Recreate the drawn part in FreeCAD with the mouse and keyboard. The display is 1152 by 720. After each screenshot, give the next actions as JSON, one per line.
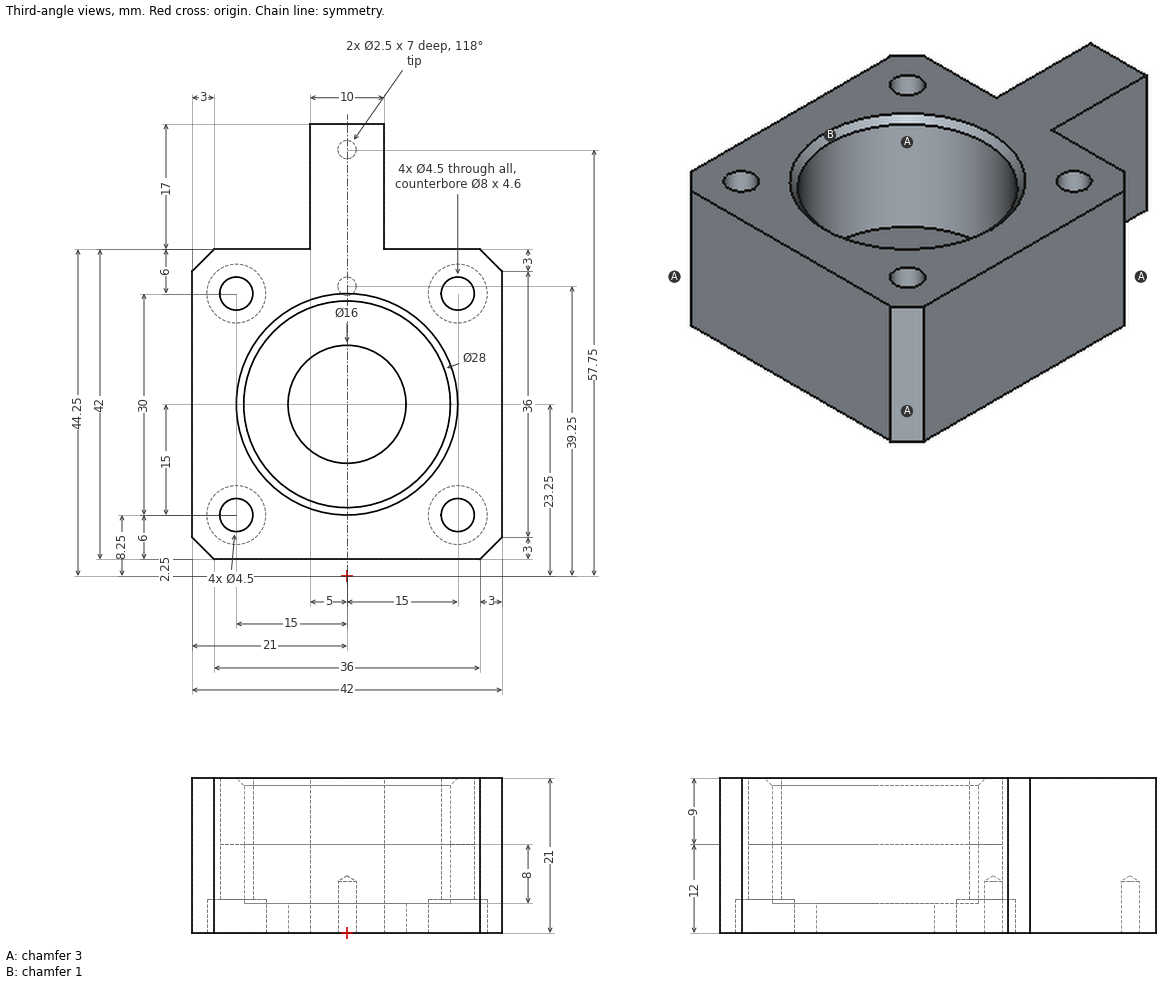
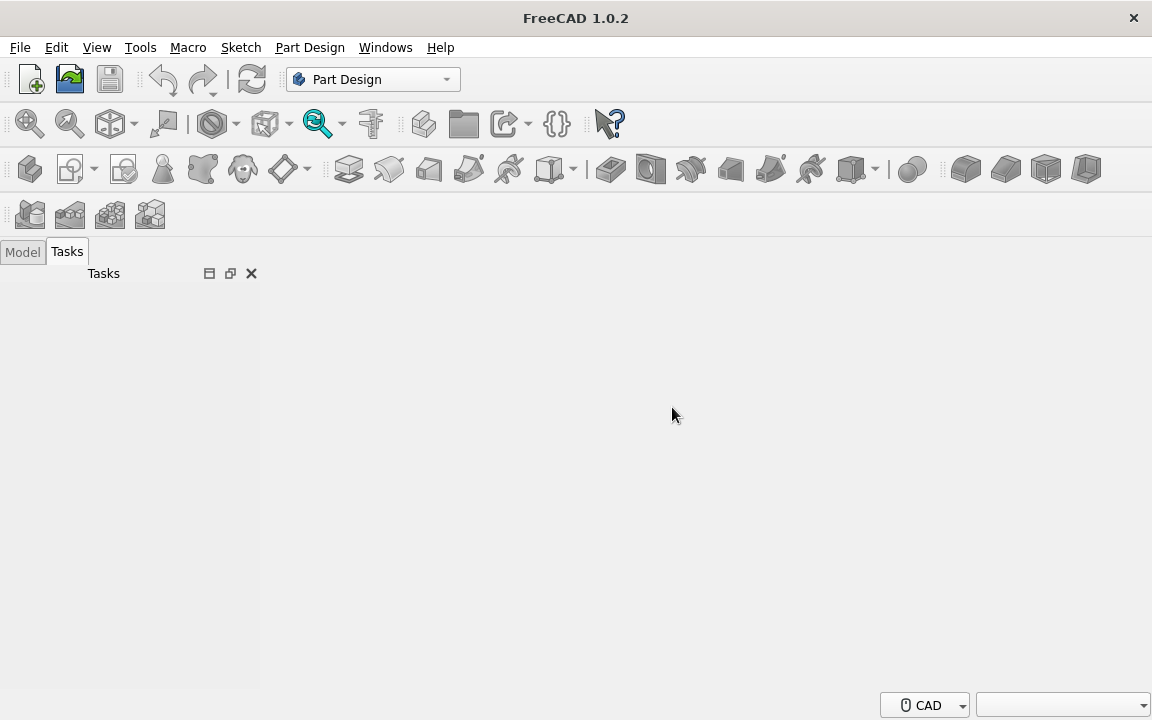
{"action": "left_click", "coordinate": [30, 80]}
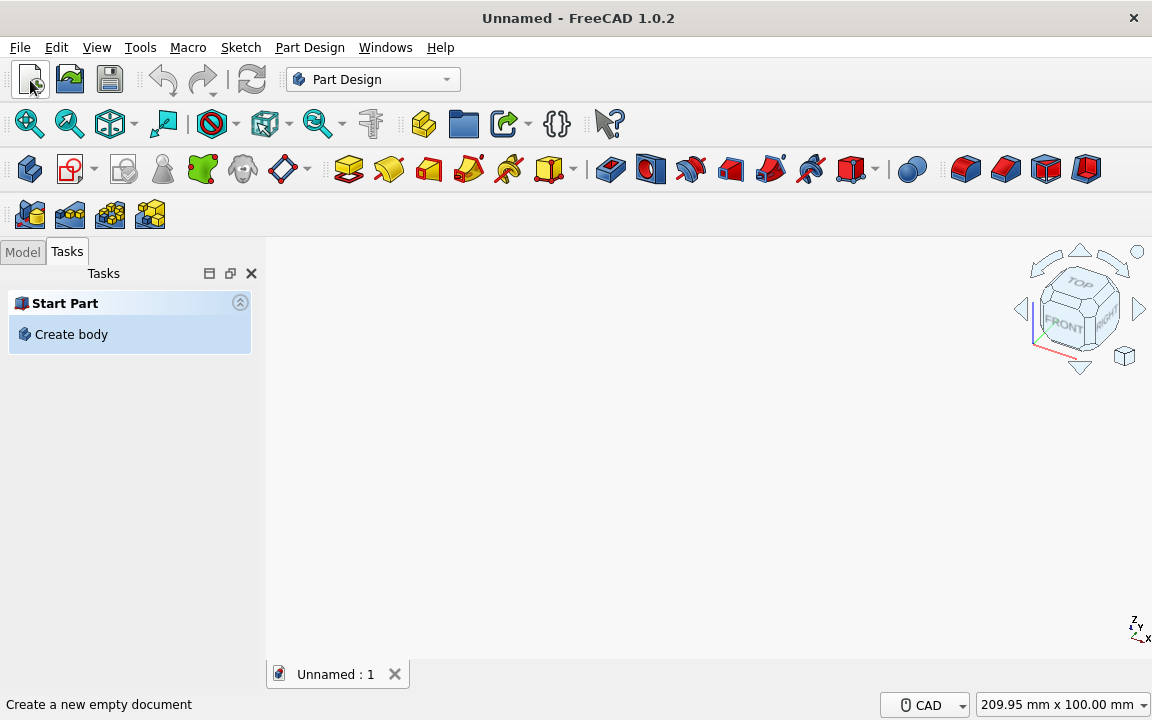
{"action": "left_click", "coordinate": [70, 170]}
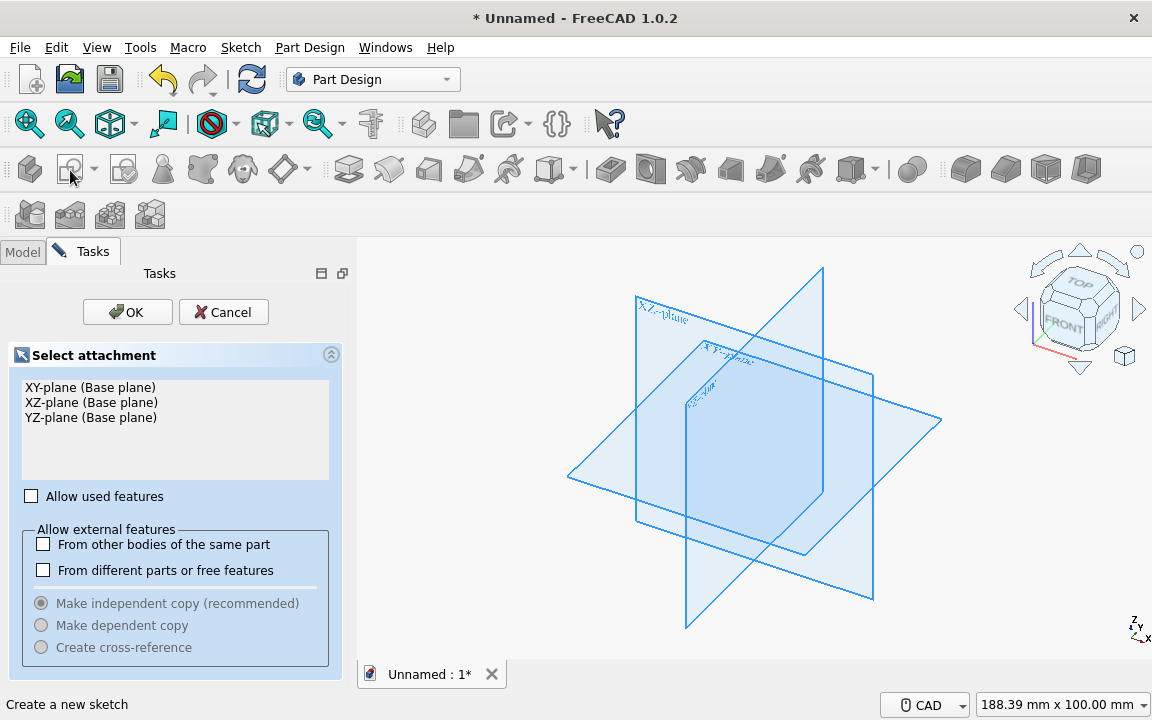
{"action": "left_click", "coordinate": [82, 388]}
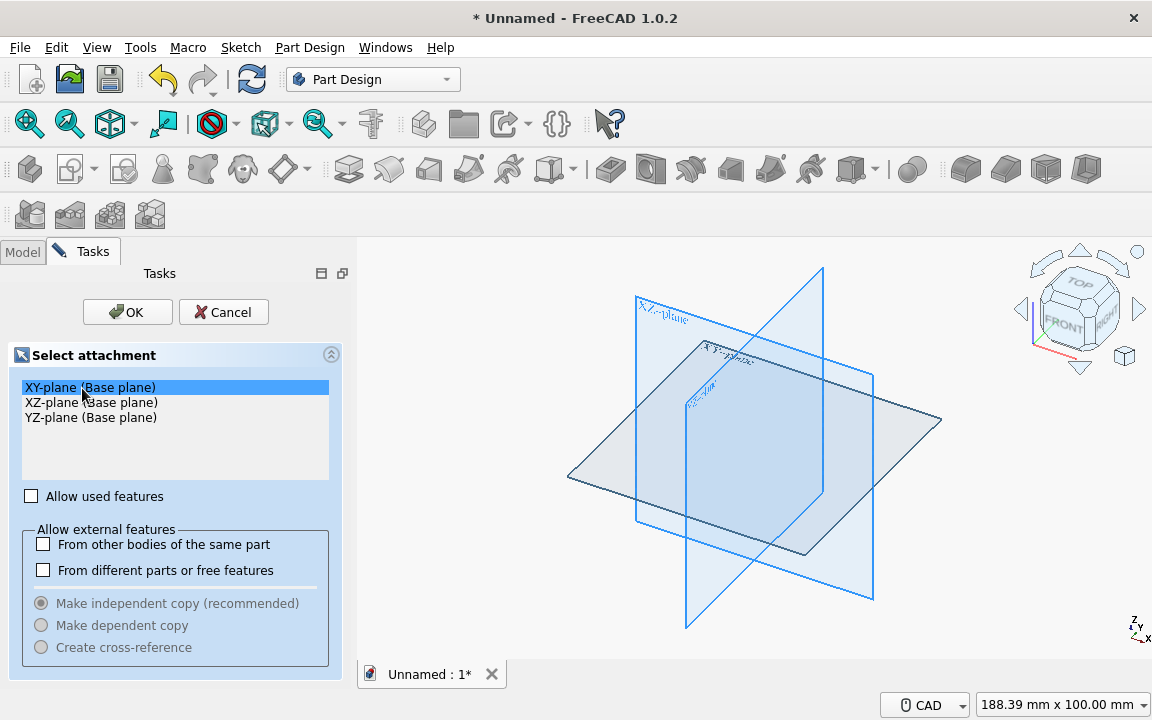
{"action": "left_click", "coordinate": [128, 312]}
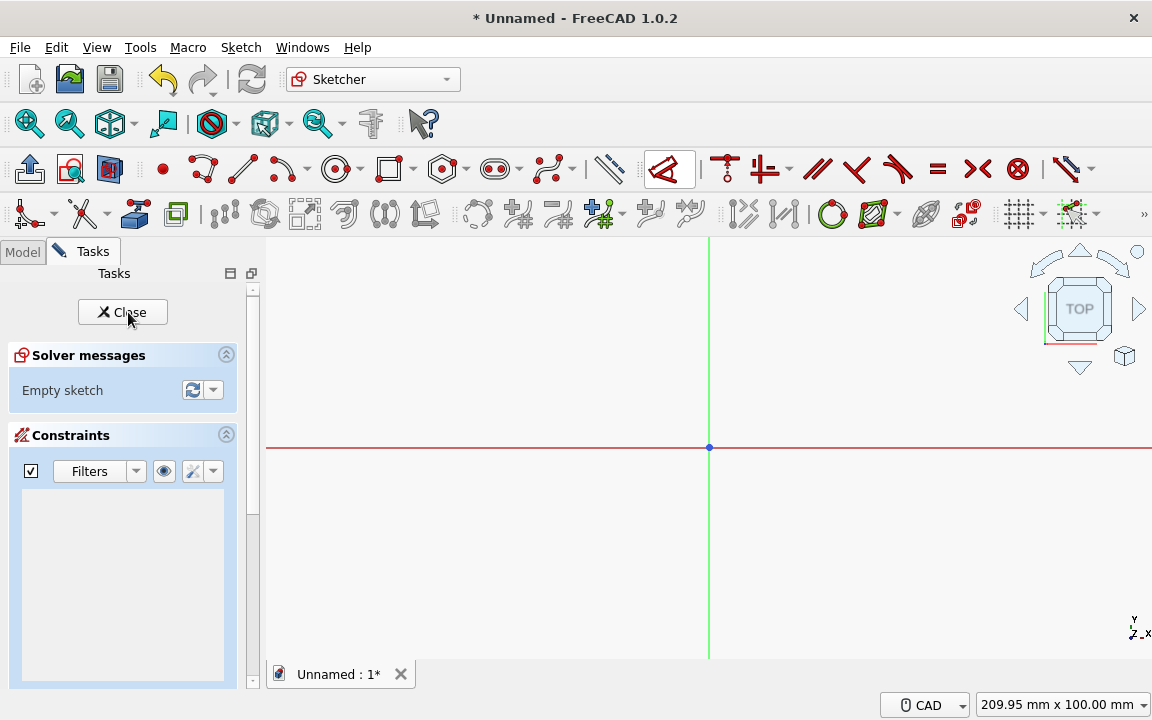
{"action": "scroll", "coordinate": [331, 631], "scroll_direction": "down", "scroll_amount": 1}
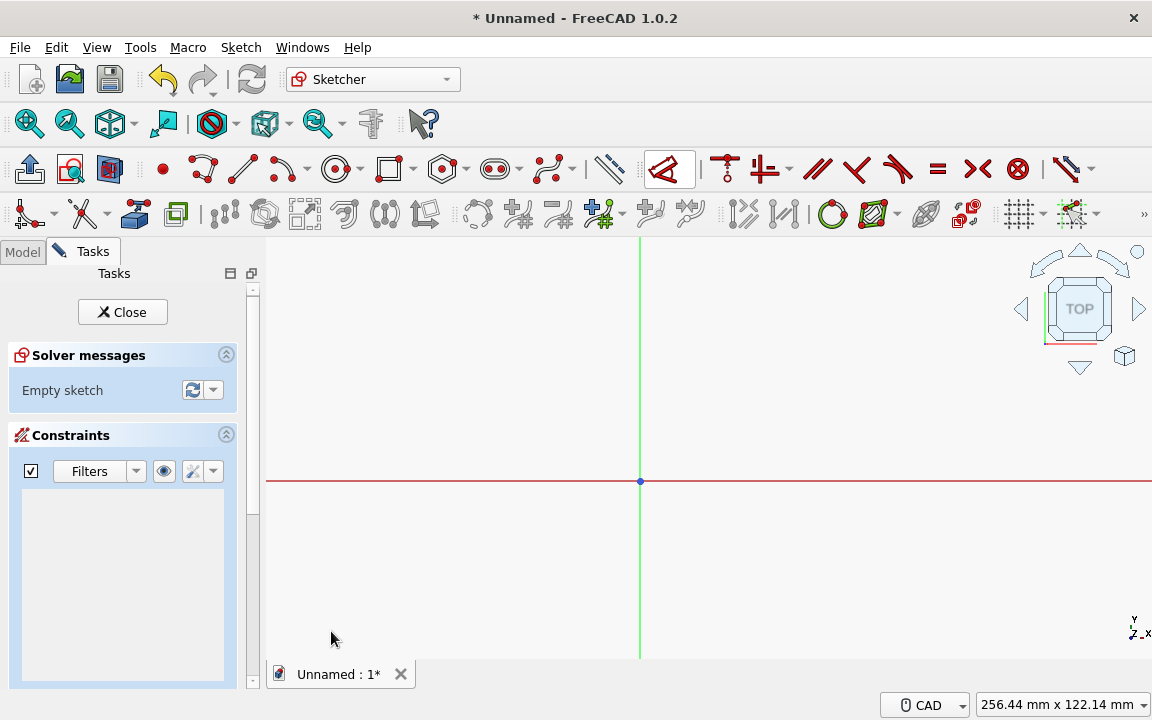
{"action": "scroll", "coordinate": [640, 352], "scroll_direction": "up", "scroll_amount": 3}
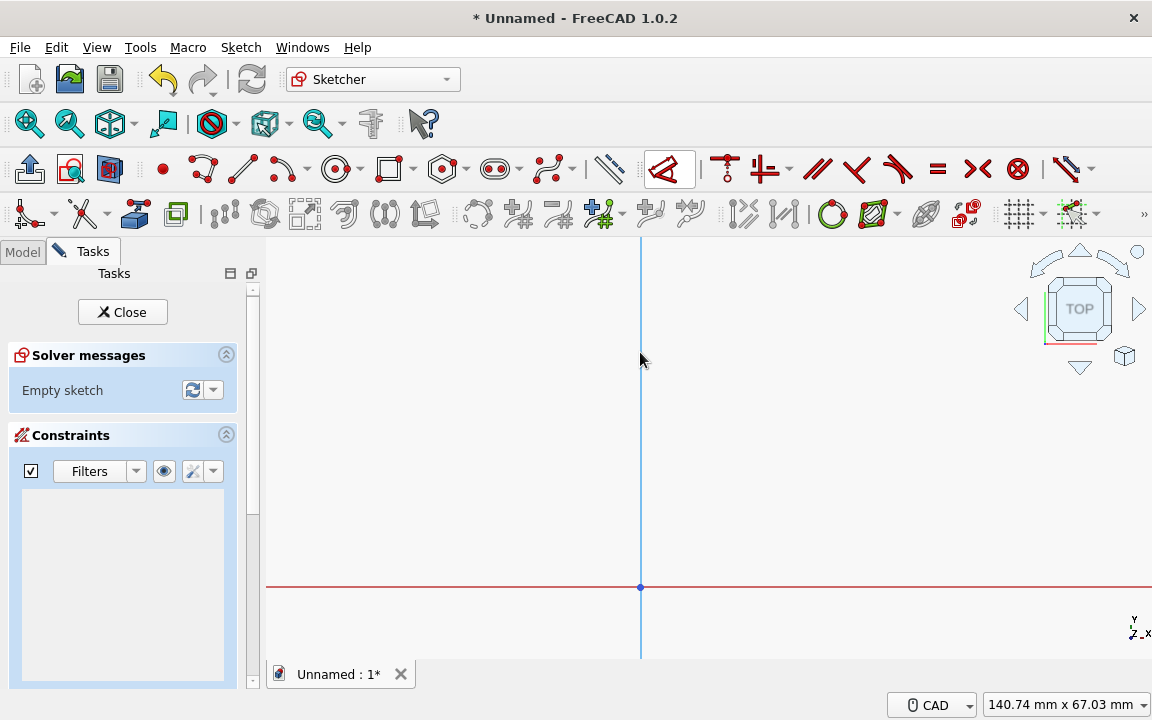
{"action": "left_click", "coordinate": [390, 170]}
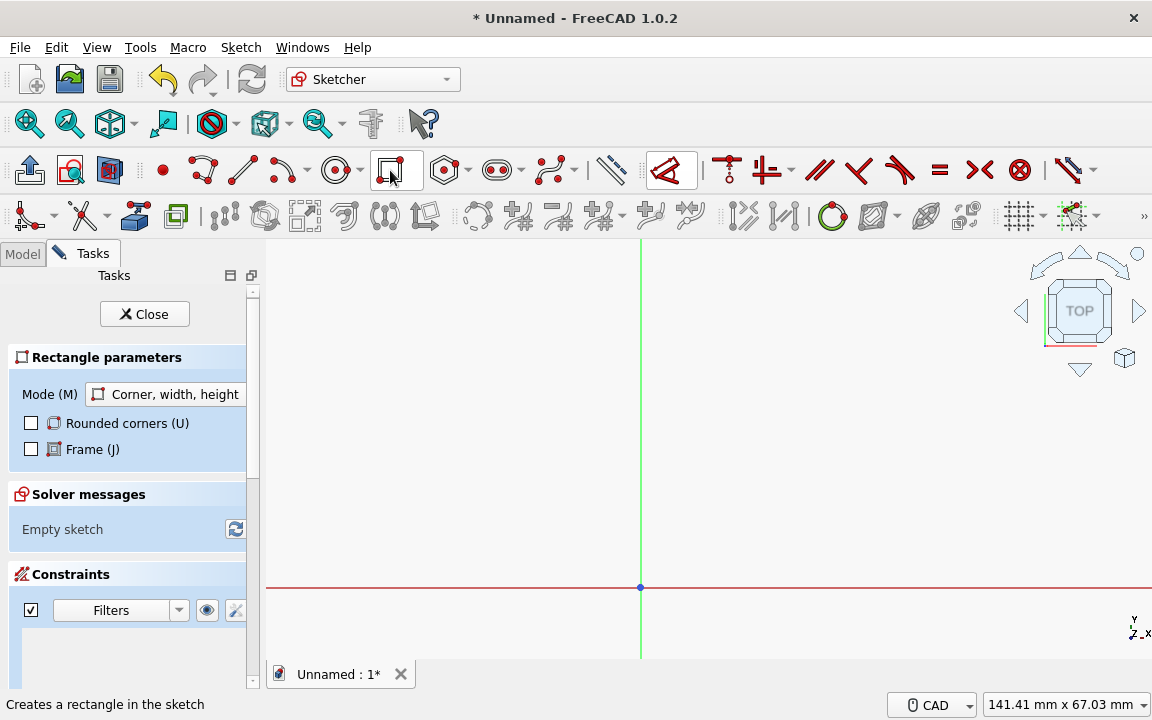
{"action": "left_click", "coordinate": [509, 311]}
{"action": "left_click", "coordinate": [772, 574]}
{"action": "key", "text": "Escape"}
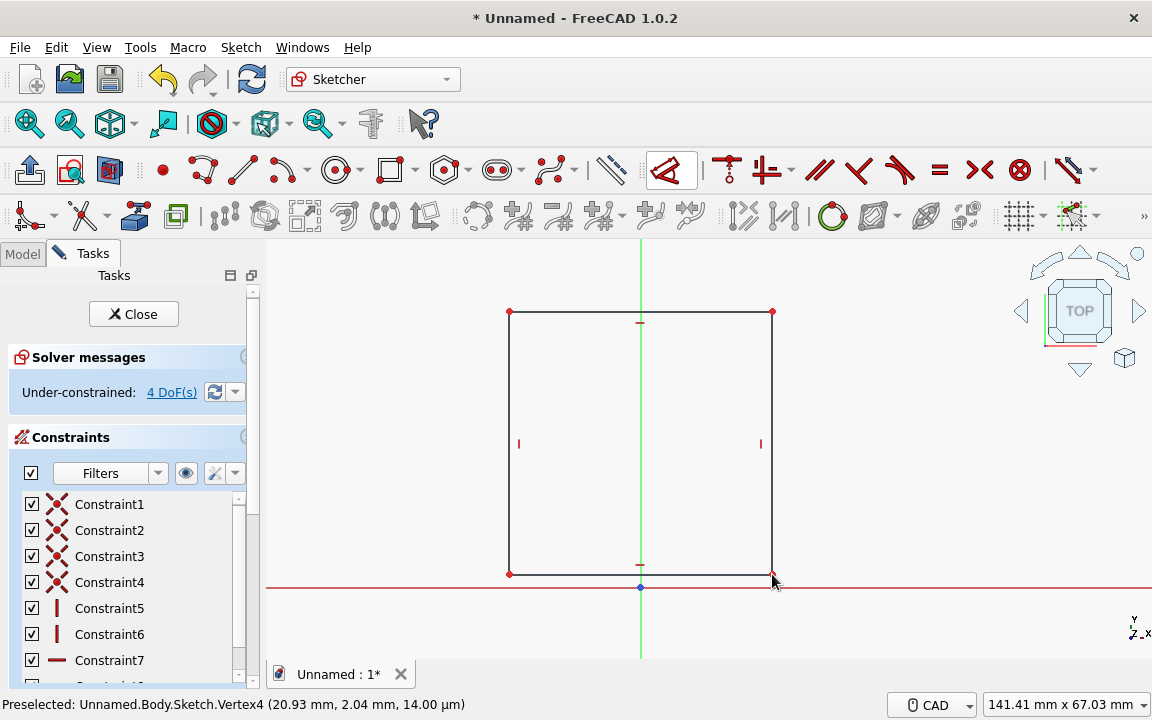
{"action": "left_click", "coordinate": [666, 170]}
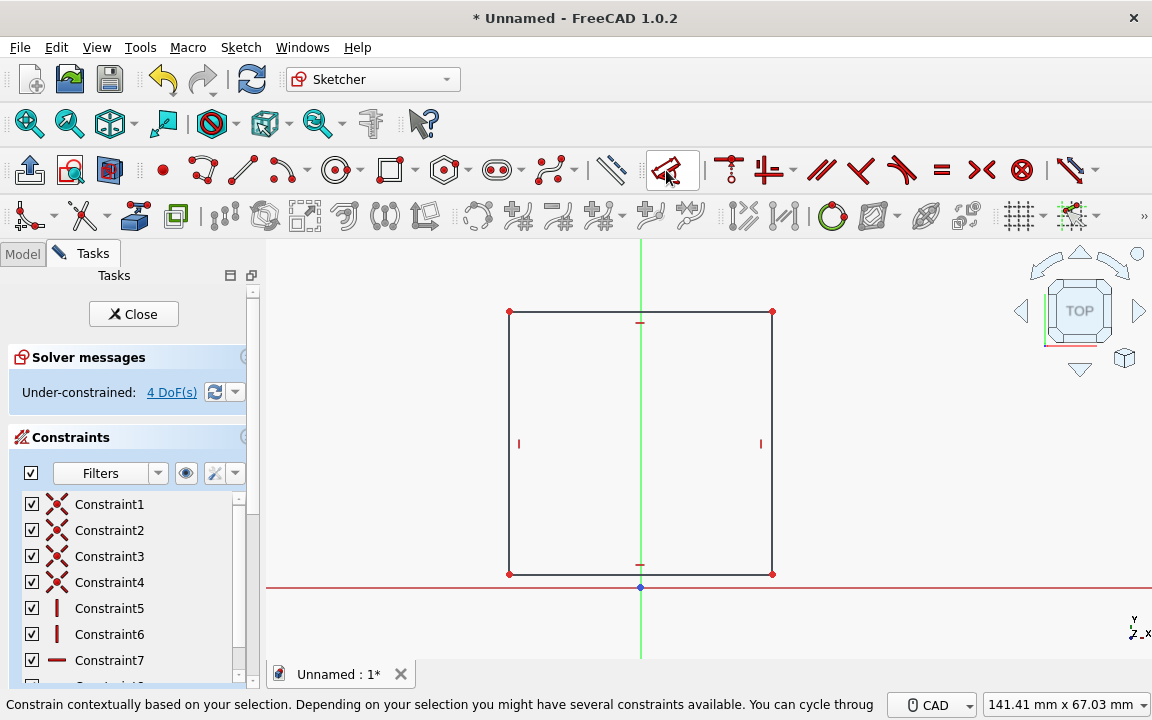
{"action": "left_click", "coordinate": [509, 391]}
{"action": "left_click", "coordinate": [475, 444]}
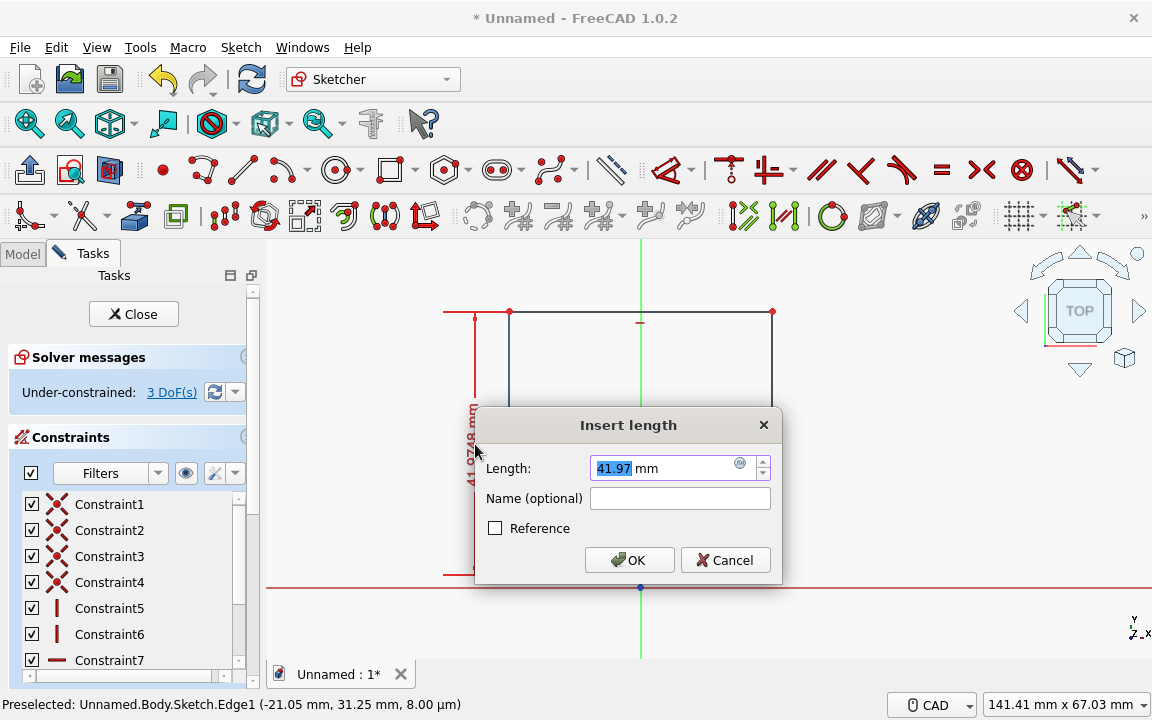
{"action": "type", "text": "42"}
{"action": "key", "text": "Return"}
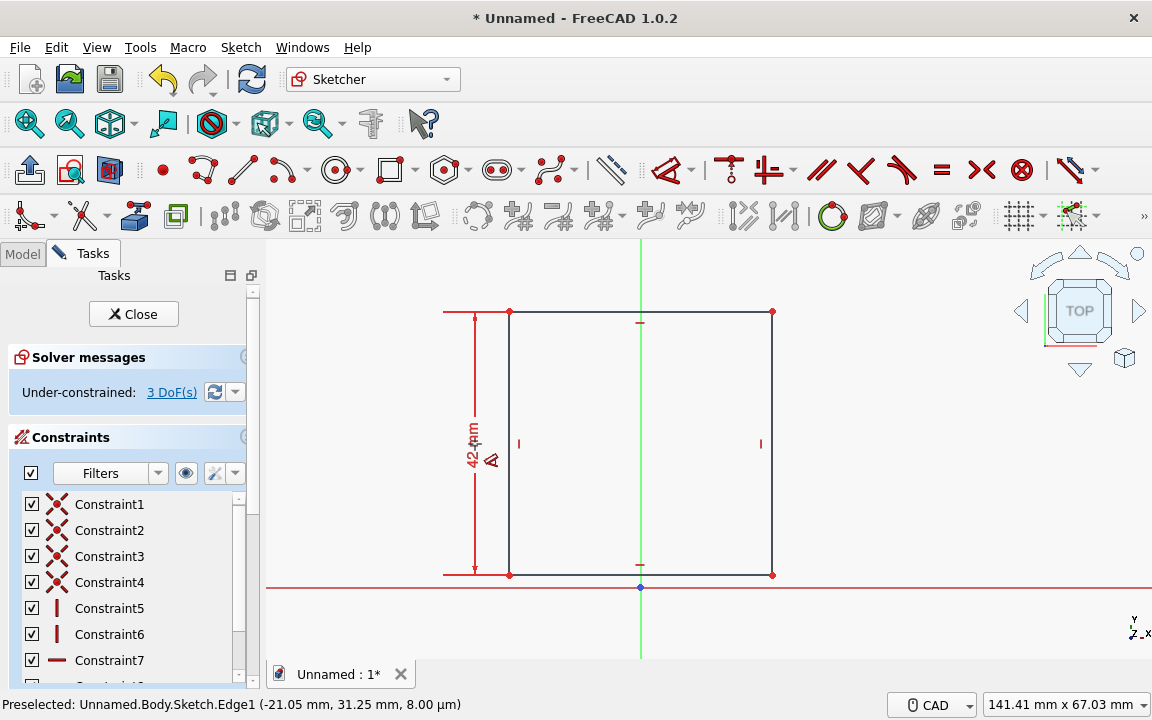
{"action": "left_click", "coordinate": [588, 575]}
{"action": "left_click", "coordinate": [580, 609]}